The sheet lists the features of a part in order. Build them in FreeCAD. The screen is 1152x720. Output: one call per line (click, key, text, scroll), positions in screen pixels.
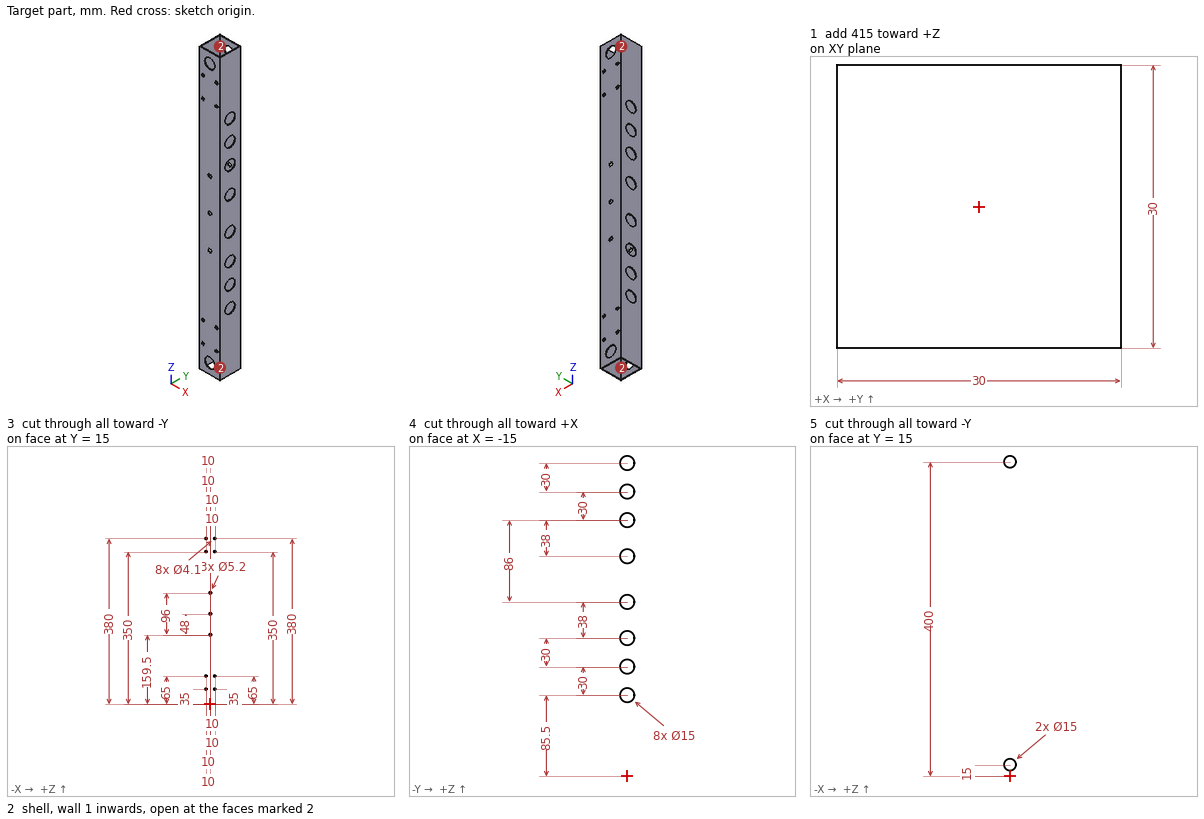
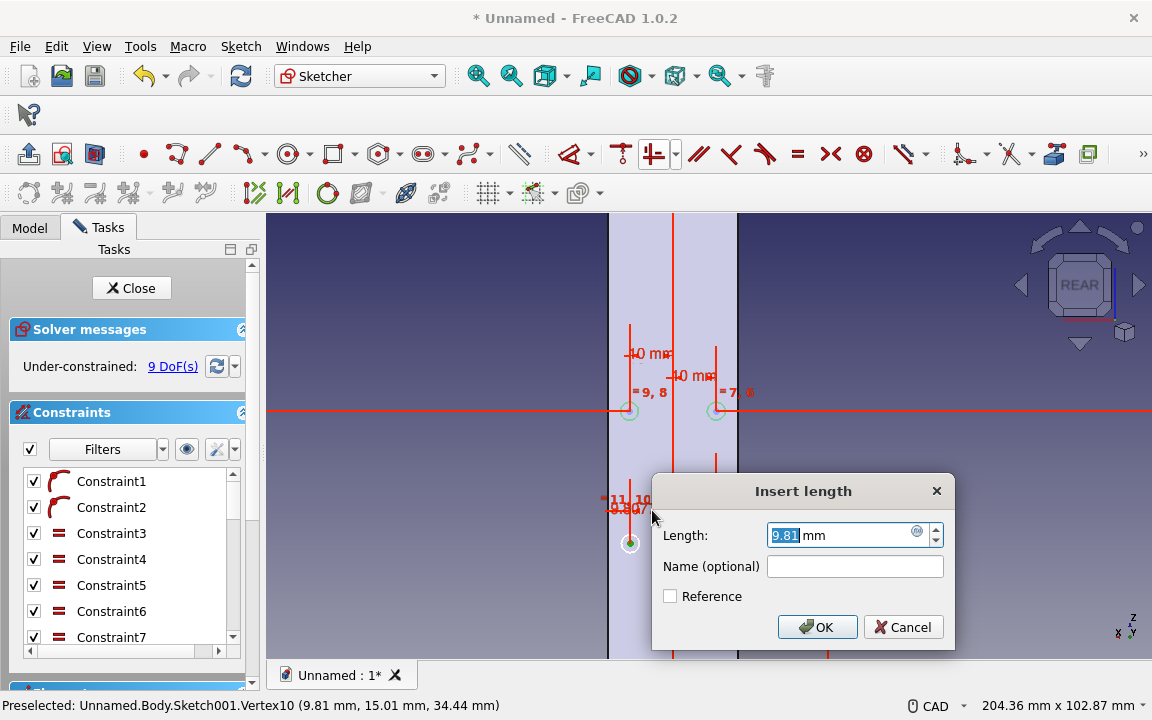
text(10)
key(Return)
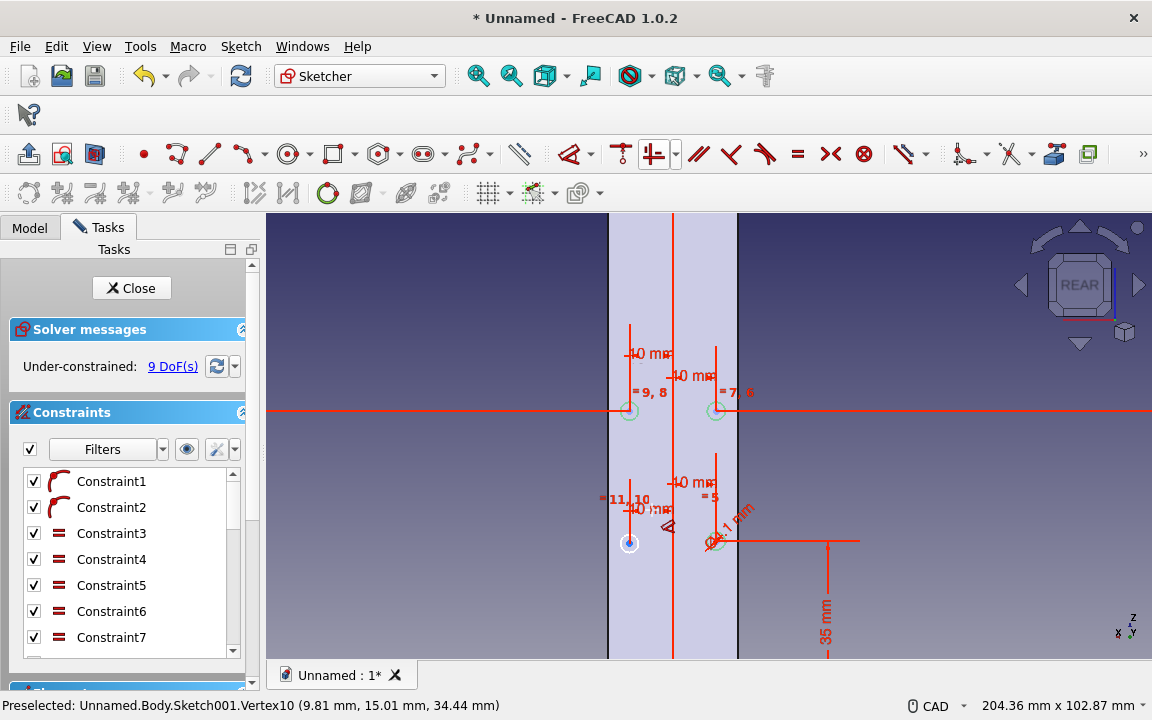
scroll(634, 549, down, 9)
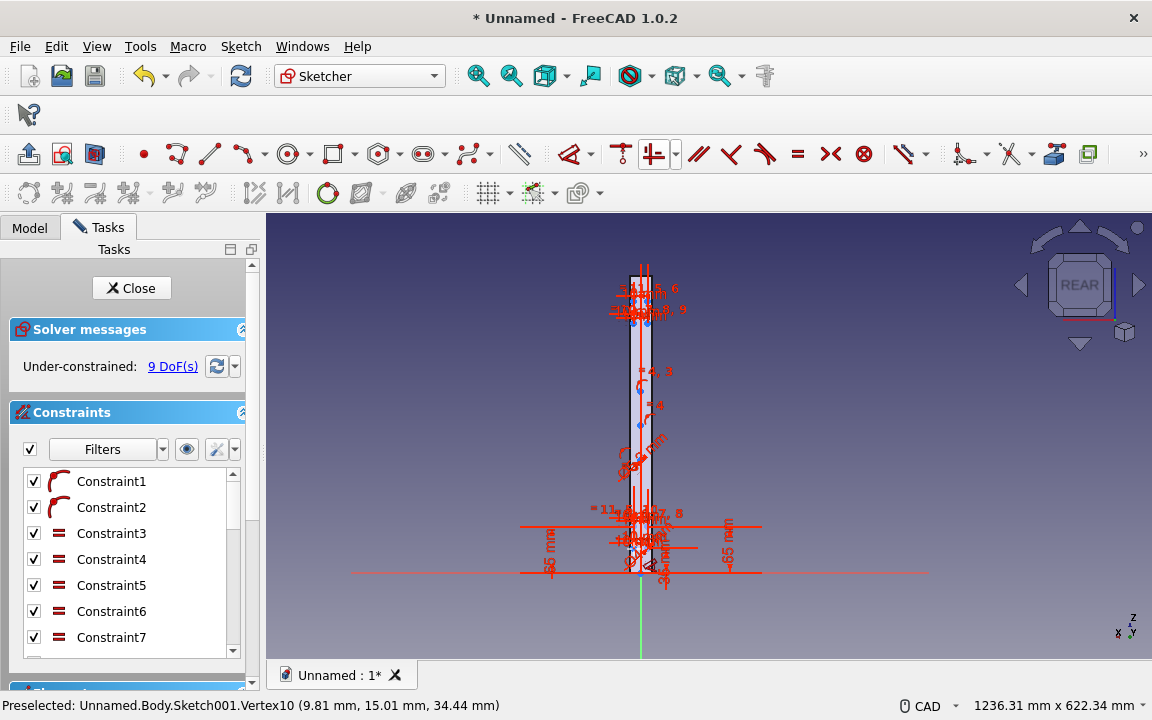
scroll(634, 549, up, 3)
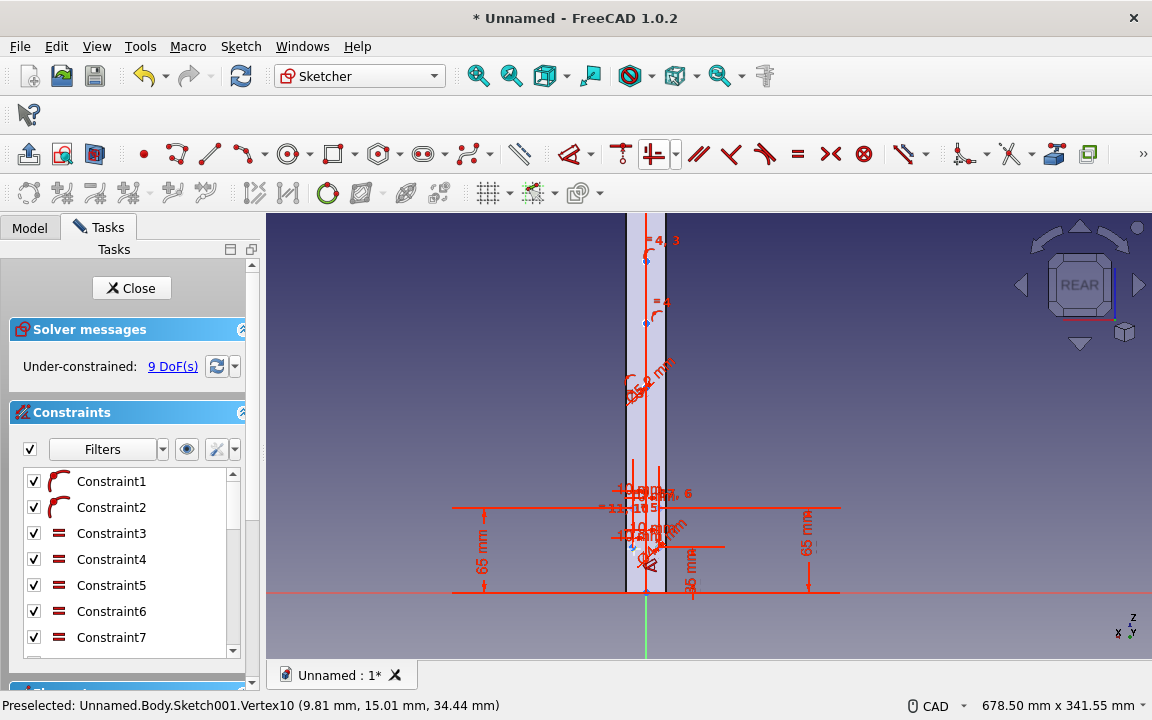
click(633, 548)
click(599, 570)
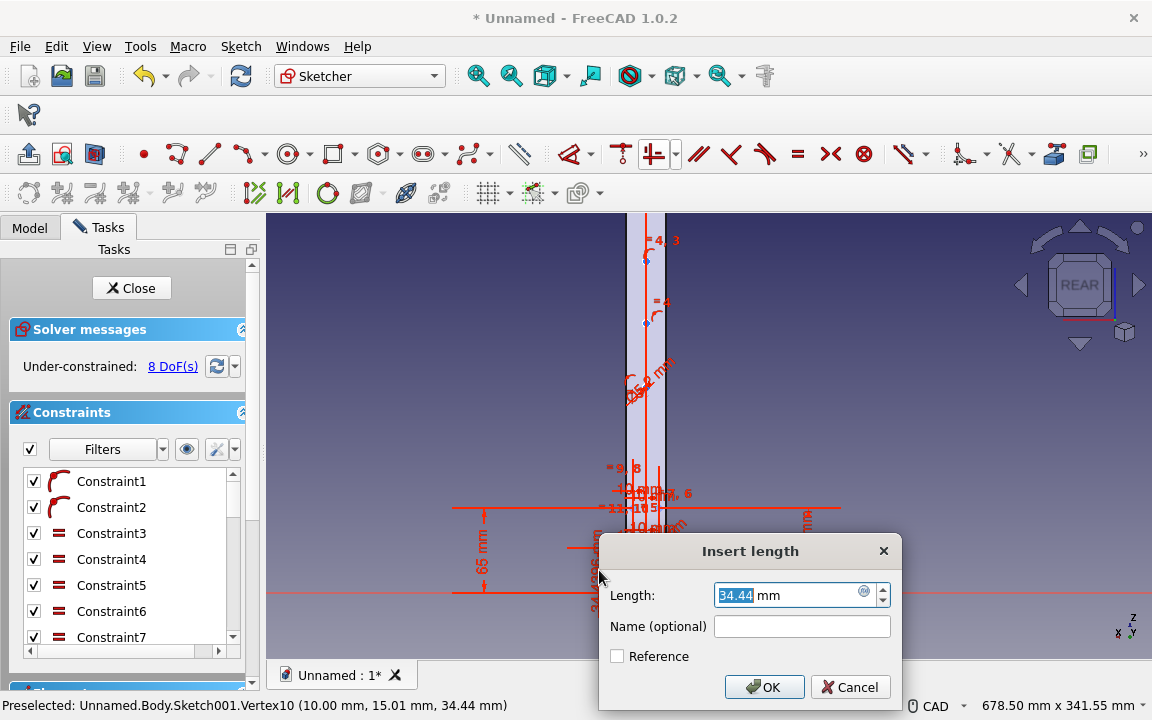
text(35)
key(Return)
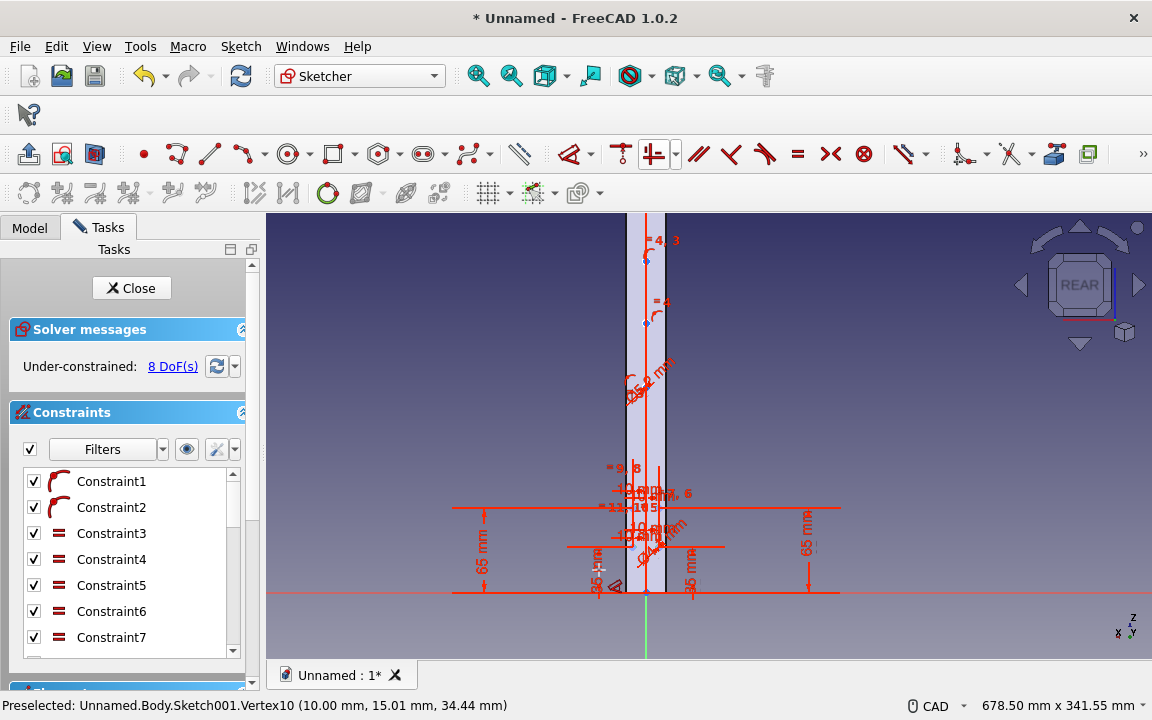
scroll(634, 549, down, 3)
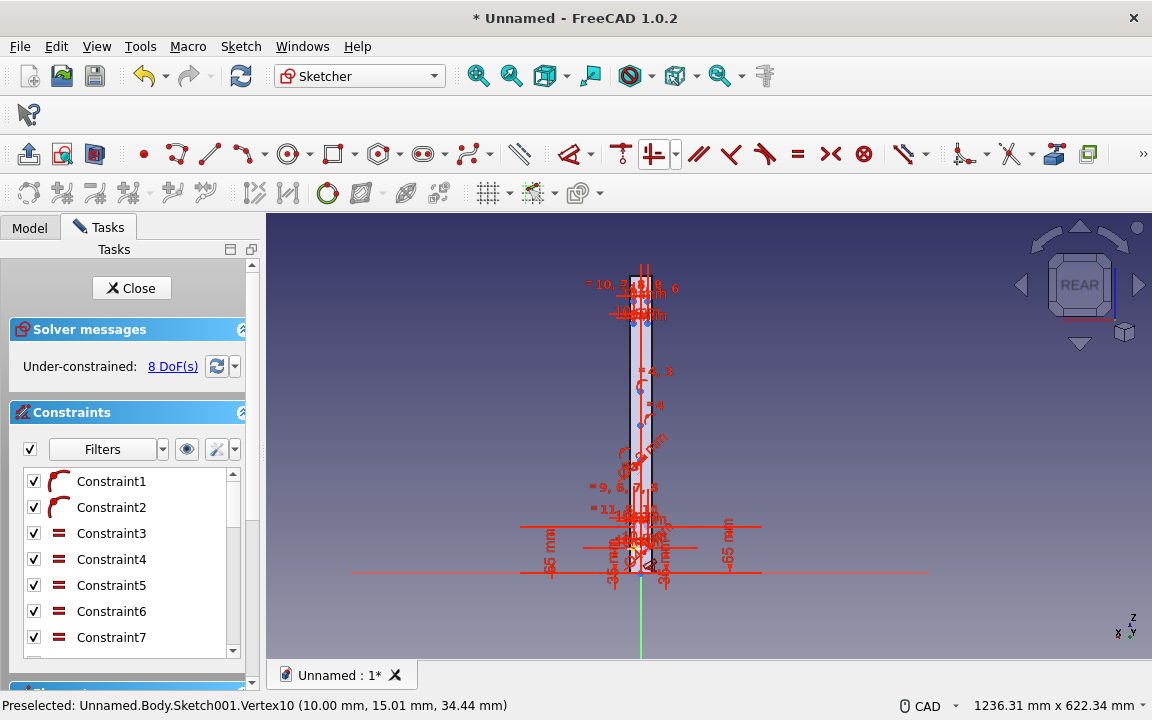
scroll(633, 302, up, 9)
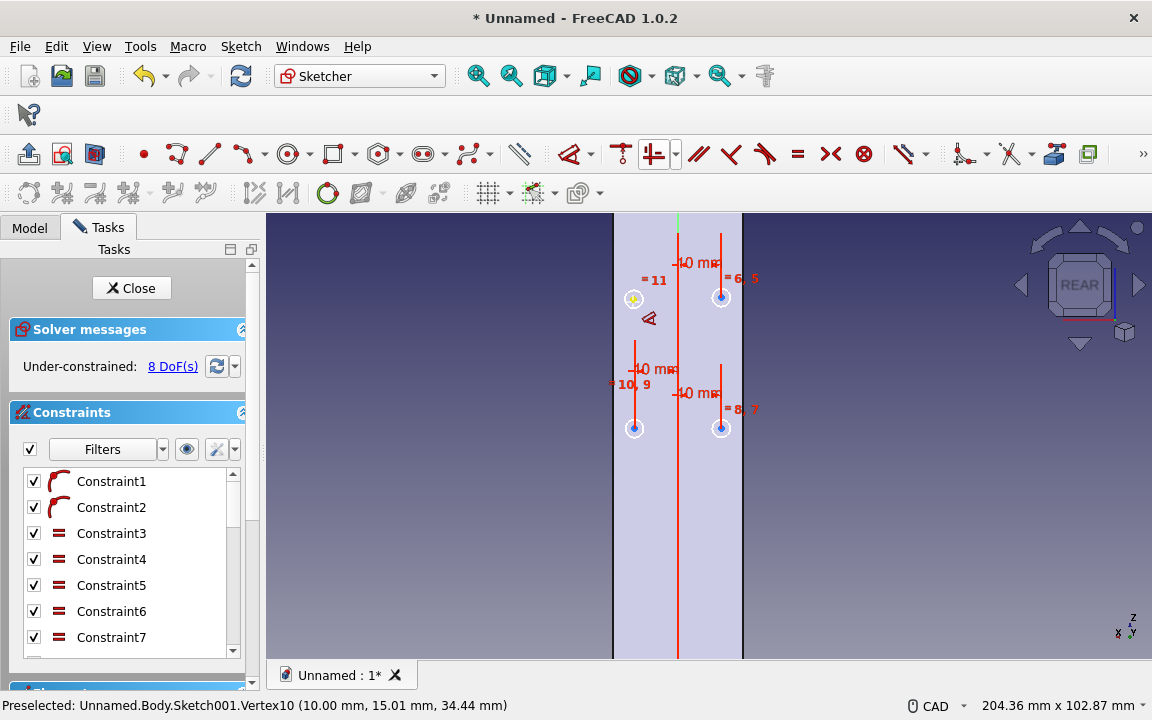
click(634, 299)
click(656, 241)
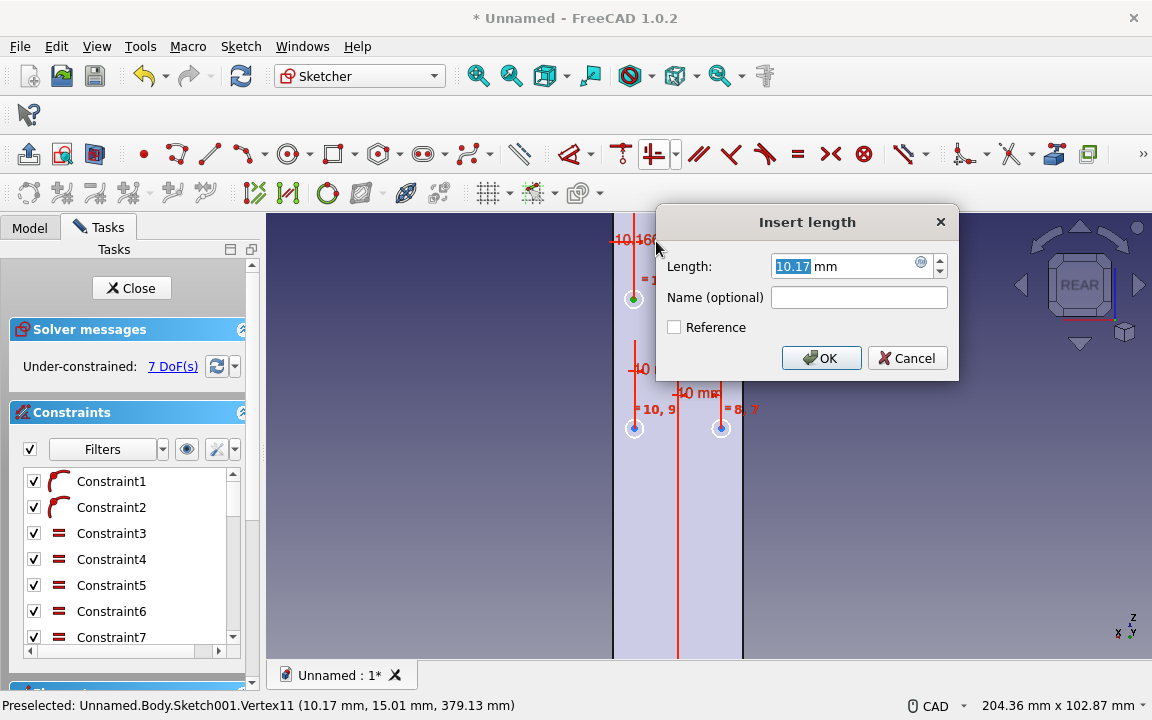
text(10)
key(Return)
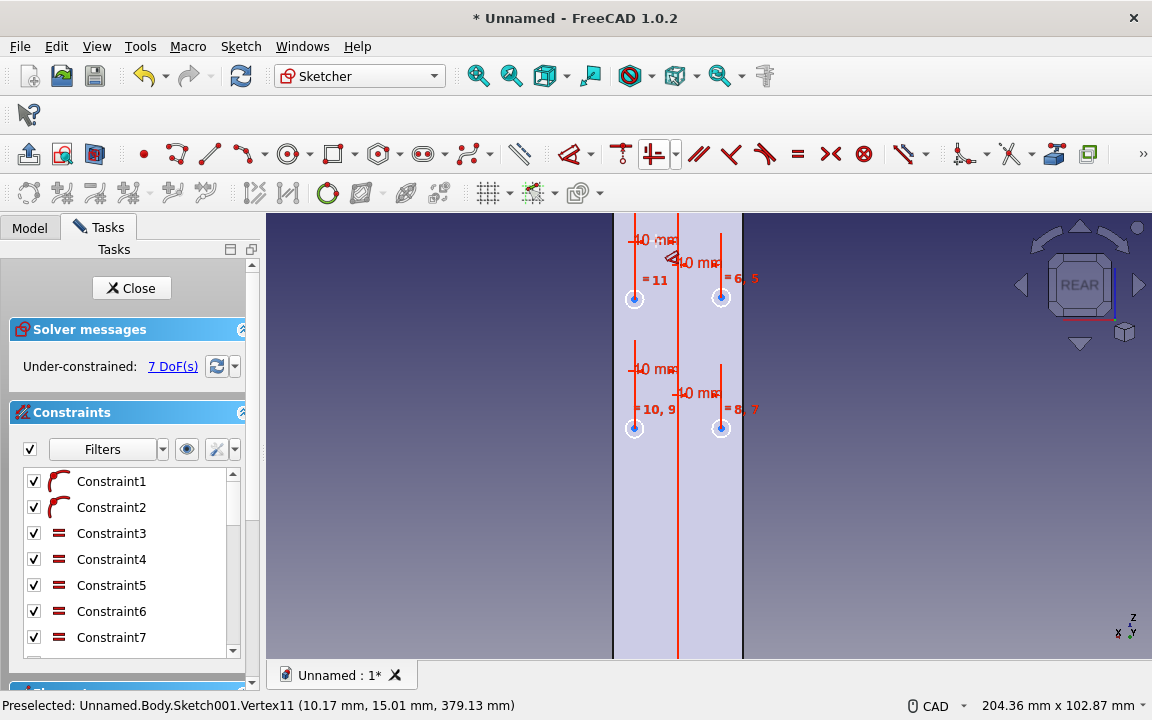
scroll(633, 302, down, 9)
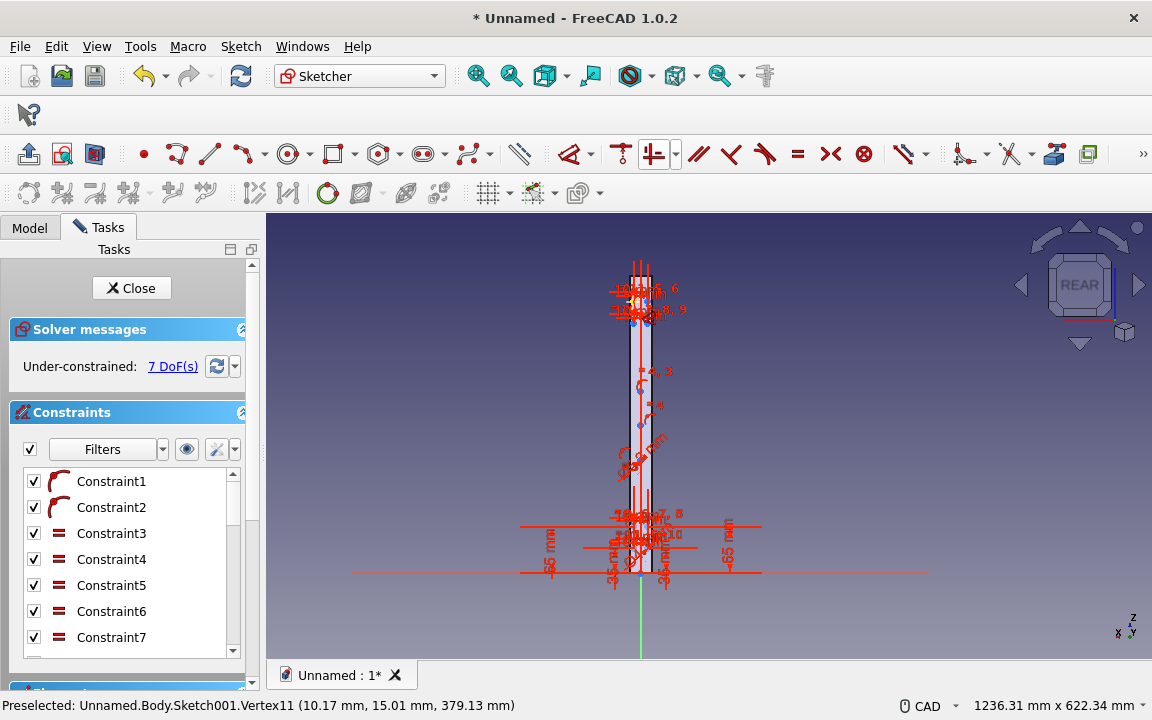
click(648, 301)
click(682, 375)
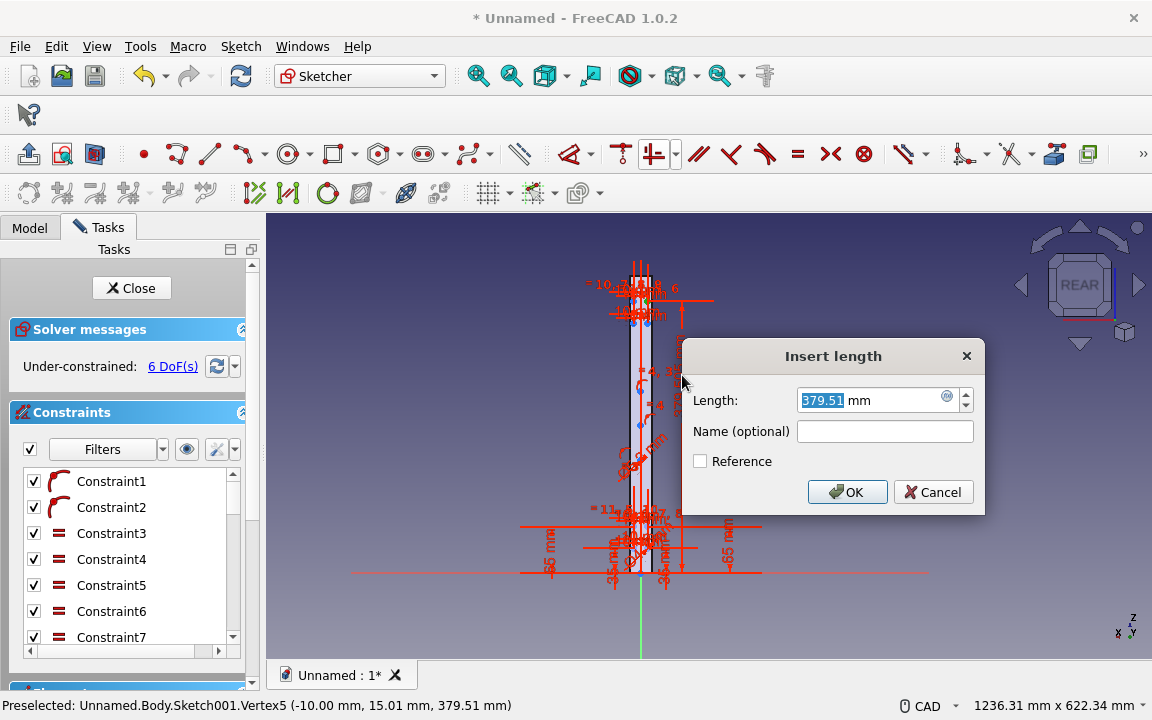
text(380)
key(Return)